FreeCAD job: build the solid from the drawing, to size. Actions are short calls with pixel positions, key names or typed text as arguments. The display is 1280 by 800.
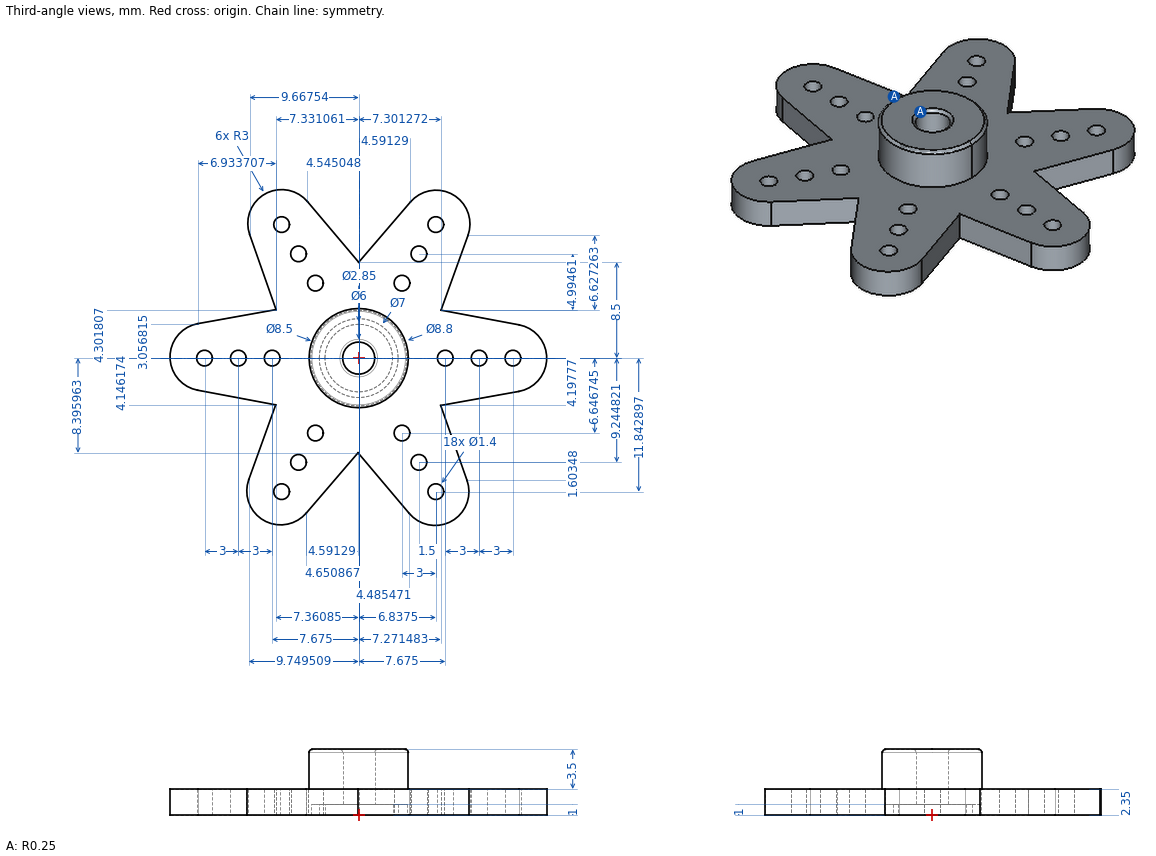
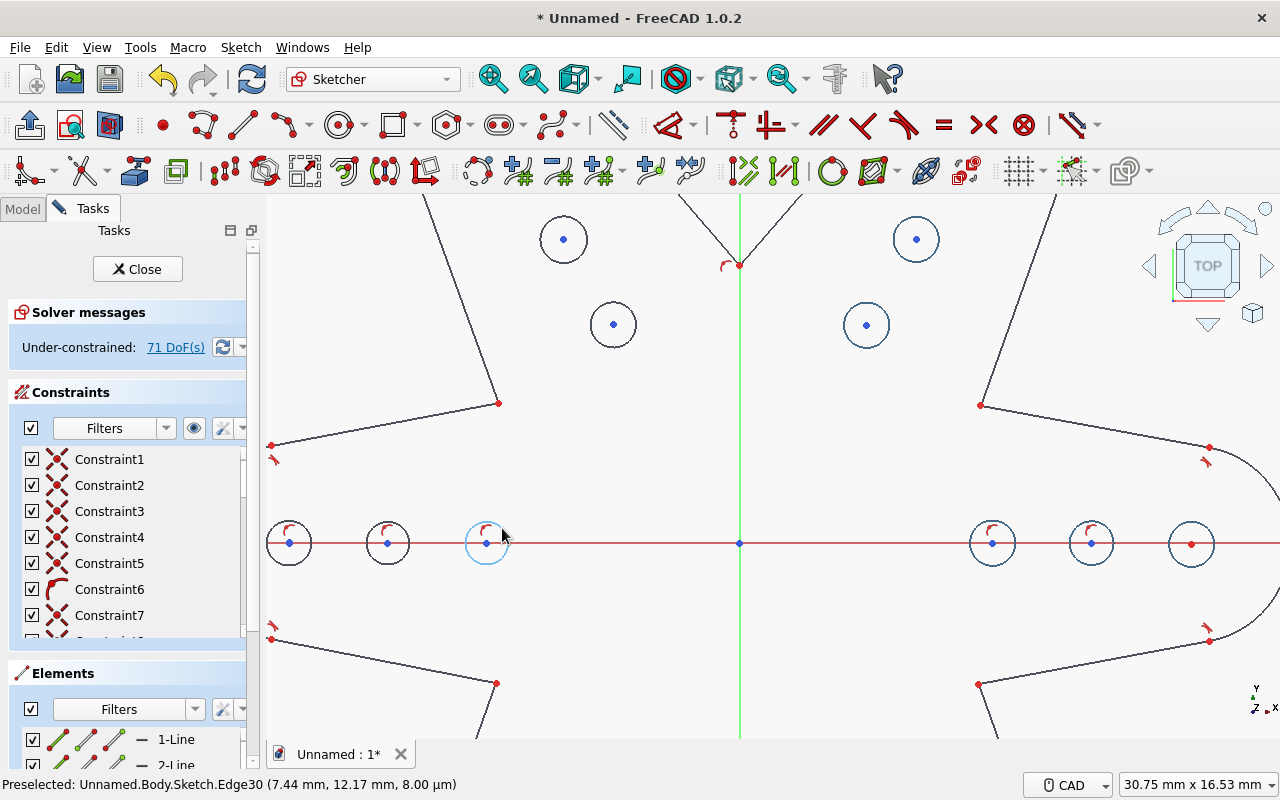
click(502, 528)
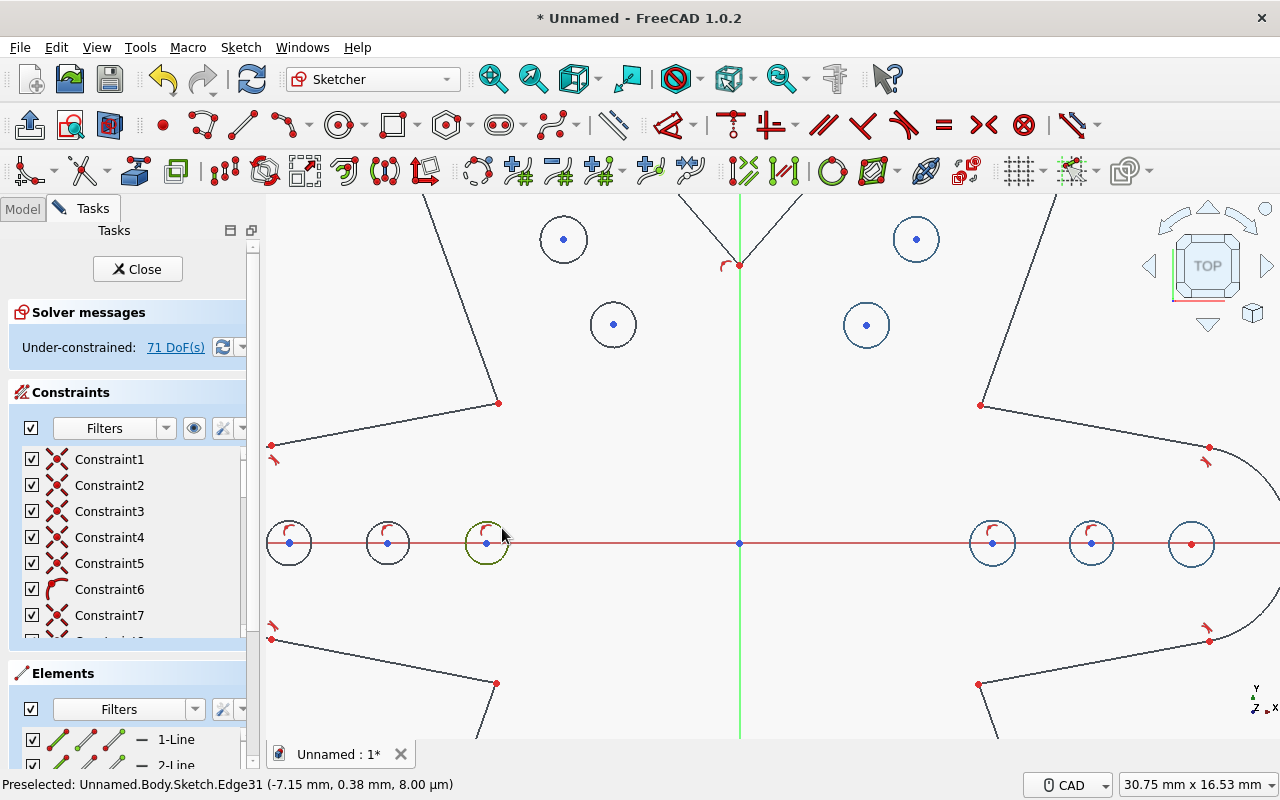
click(403, 528)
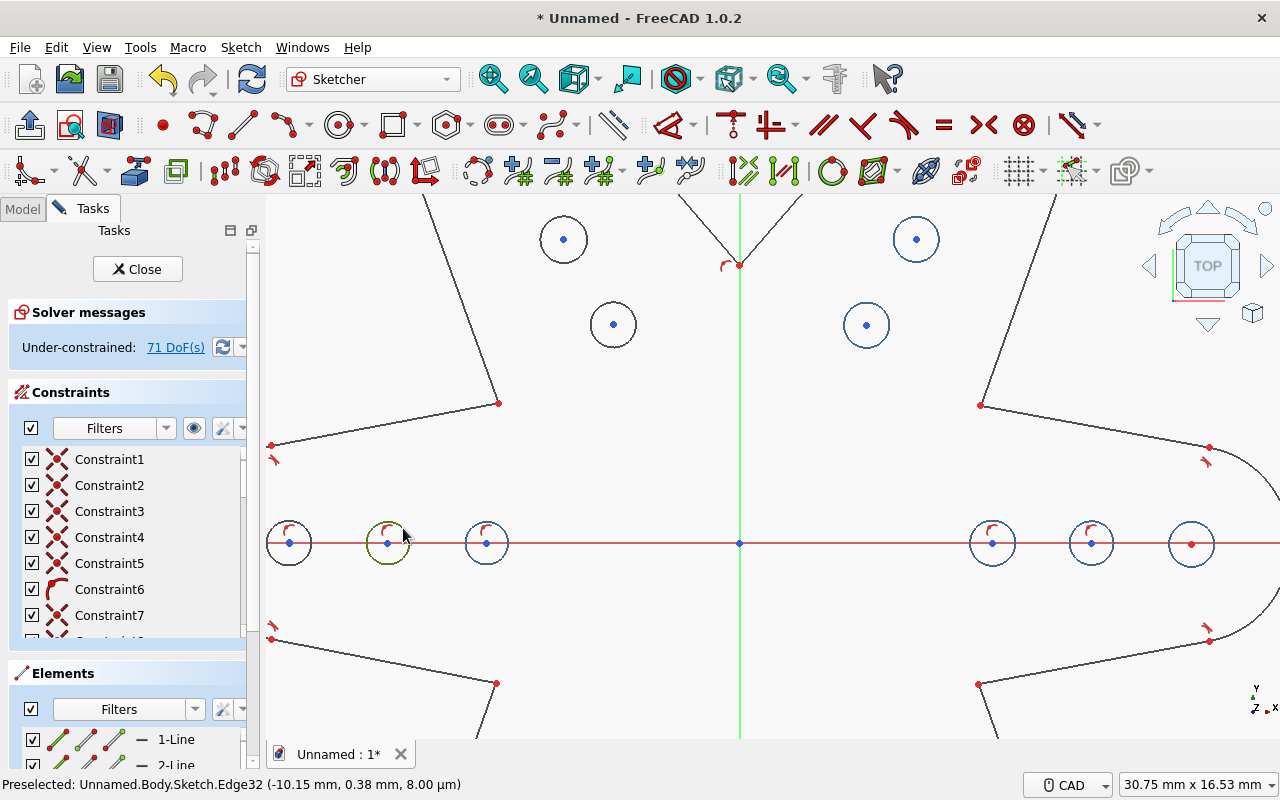
click(305, 527)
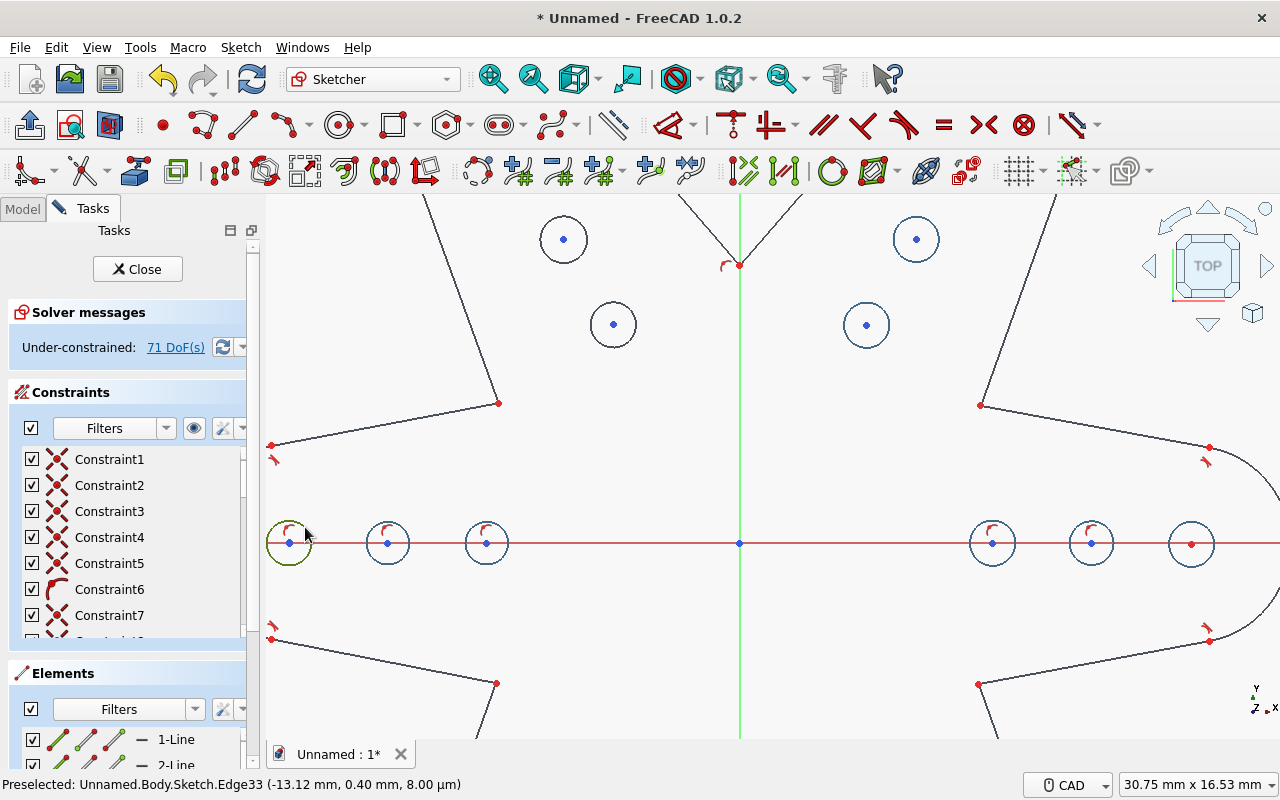
click(629, 309)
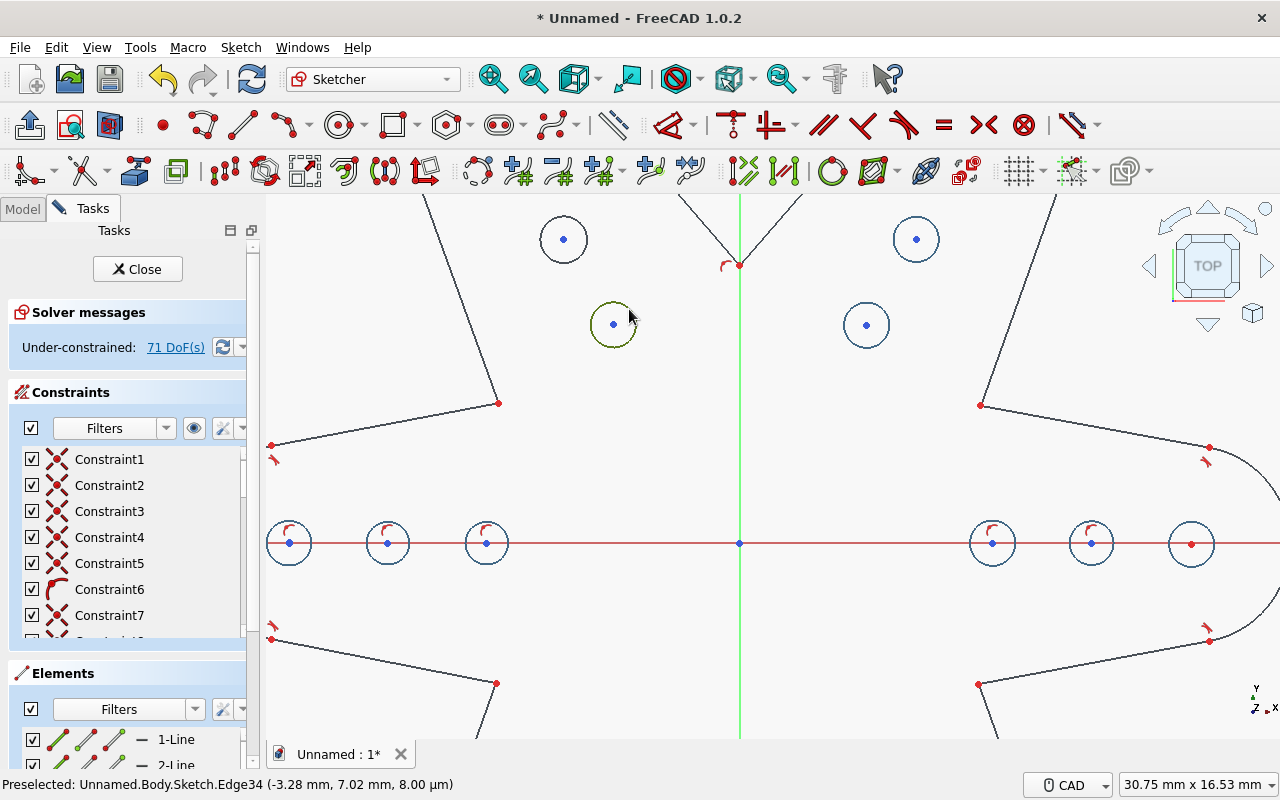
click(580, 223)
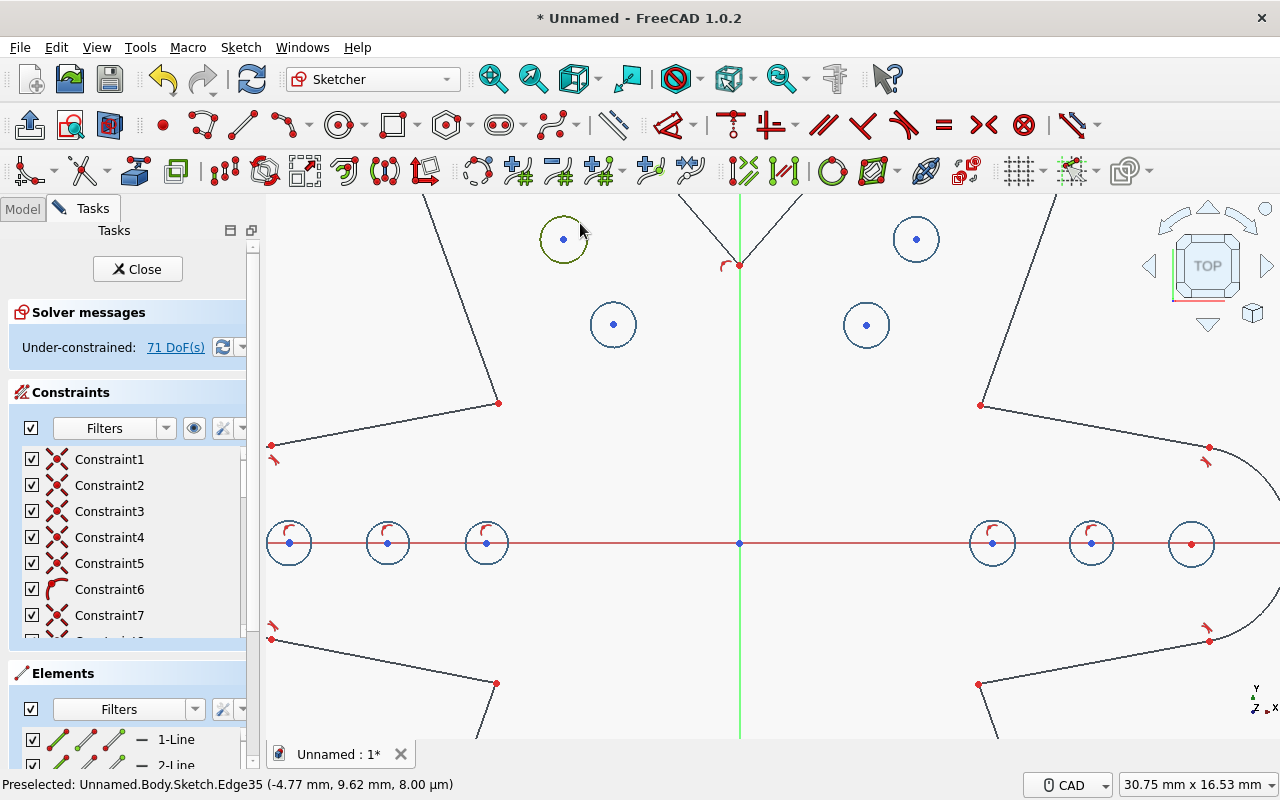
scroll(685, 423, down, 5)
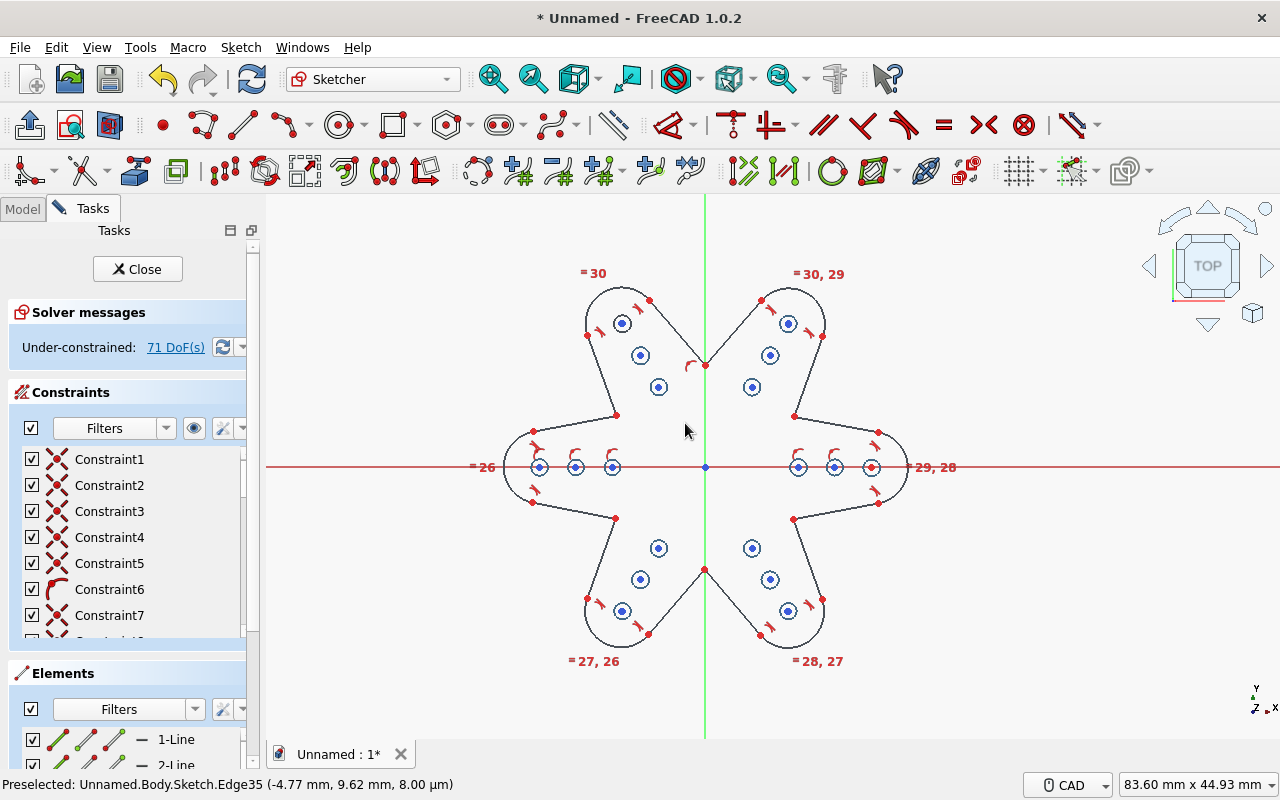
scroll(628, 318, up, 3)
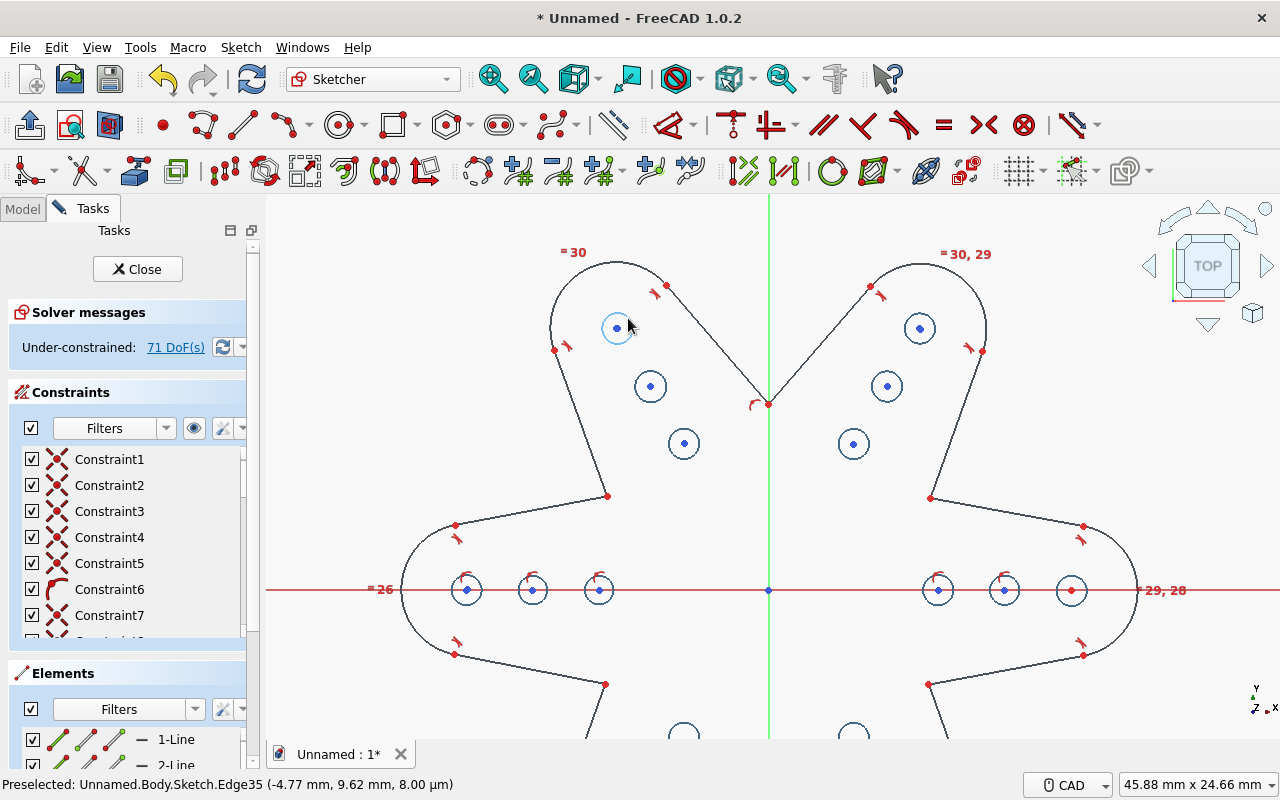
click(629, 318)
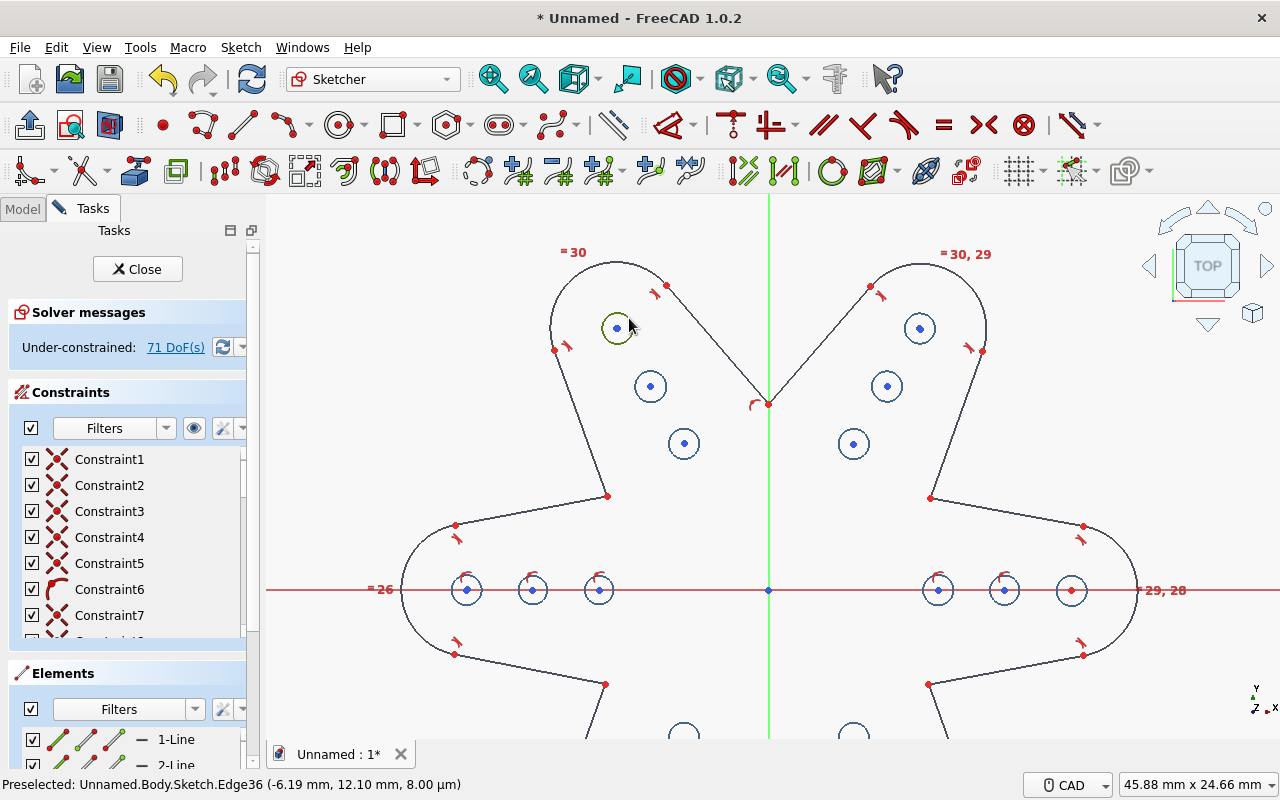
click(944, 126)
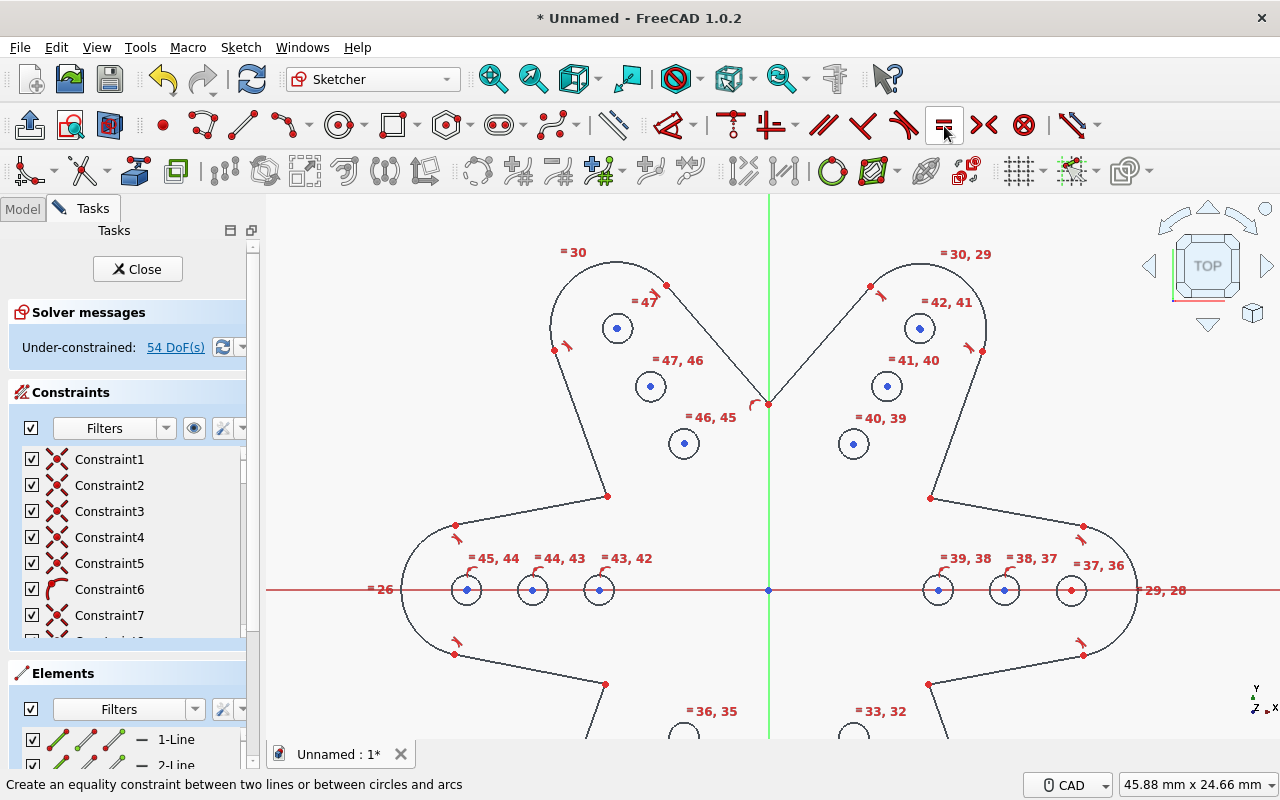
click(1072, 591)